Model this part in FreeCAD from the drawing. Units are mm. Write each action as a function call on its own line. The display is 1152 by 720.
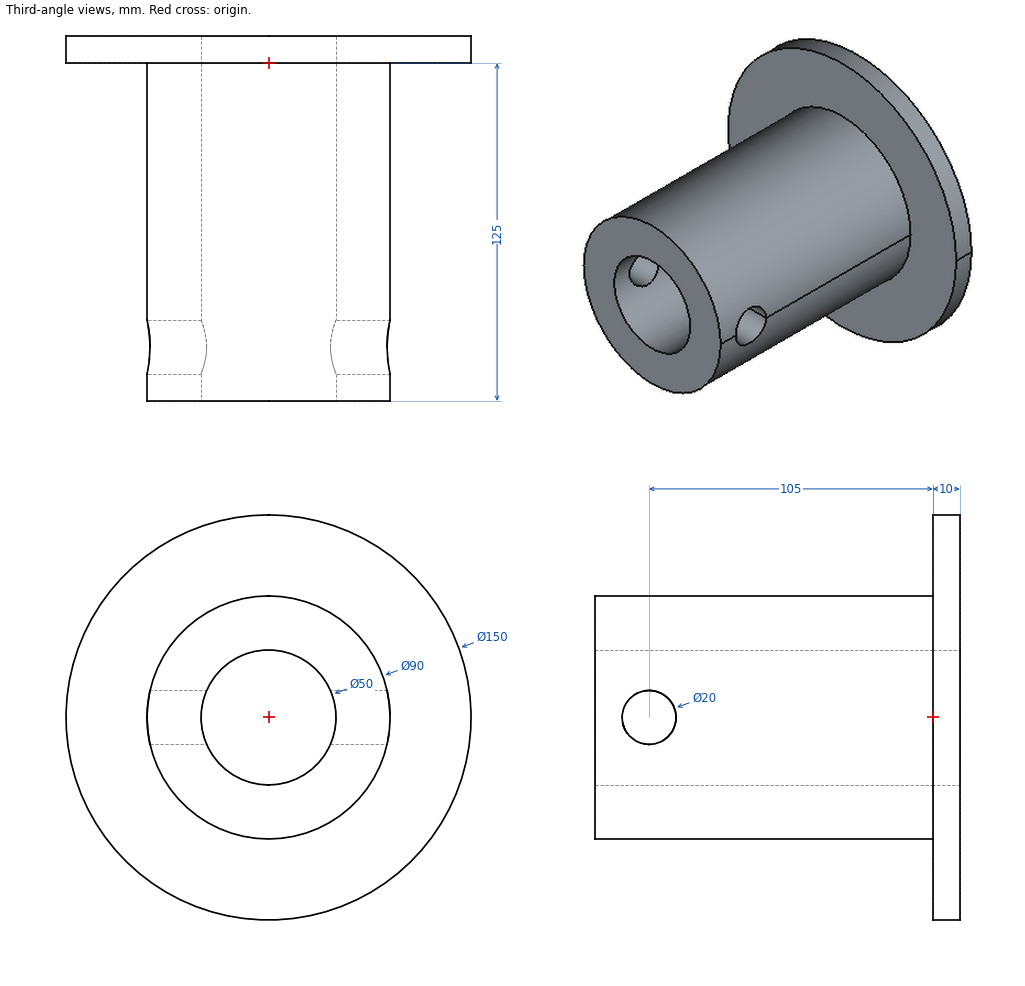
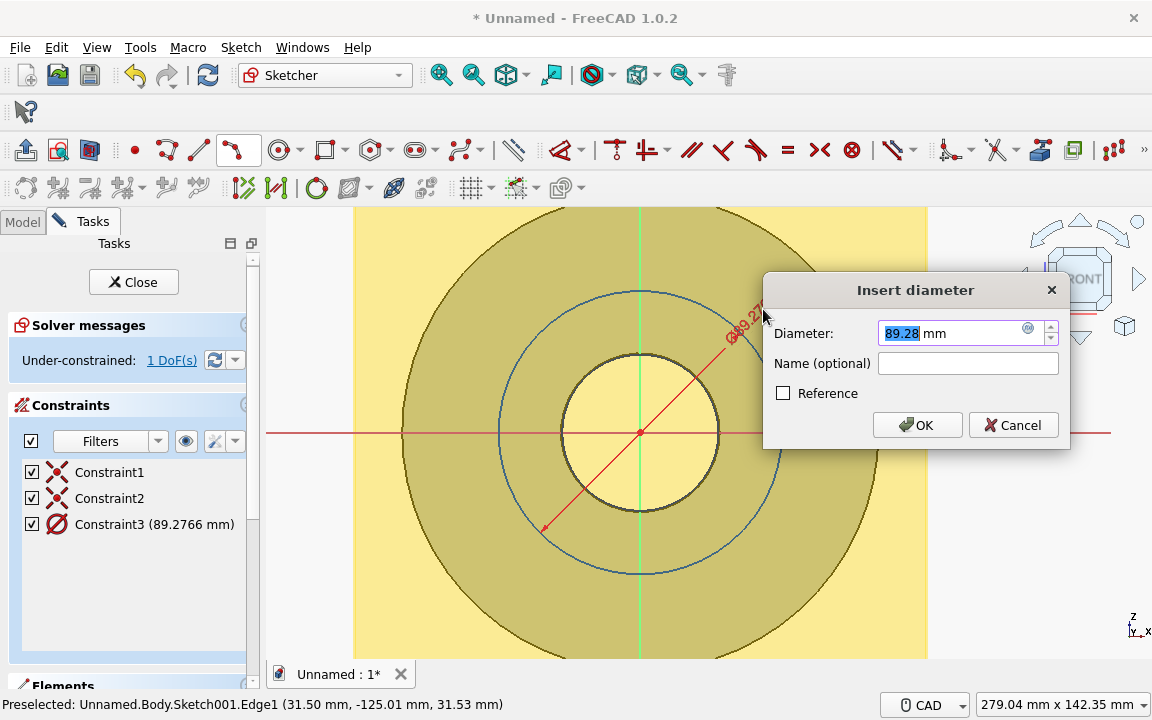
text(90)
key(Return)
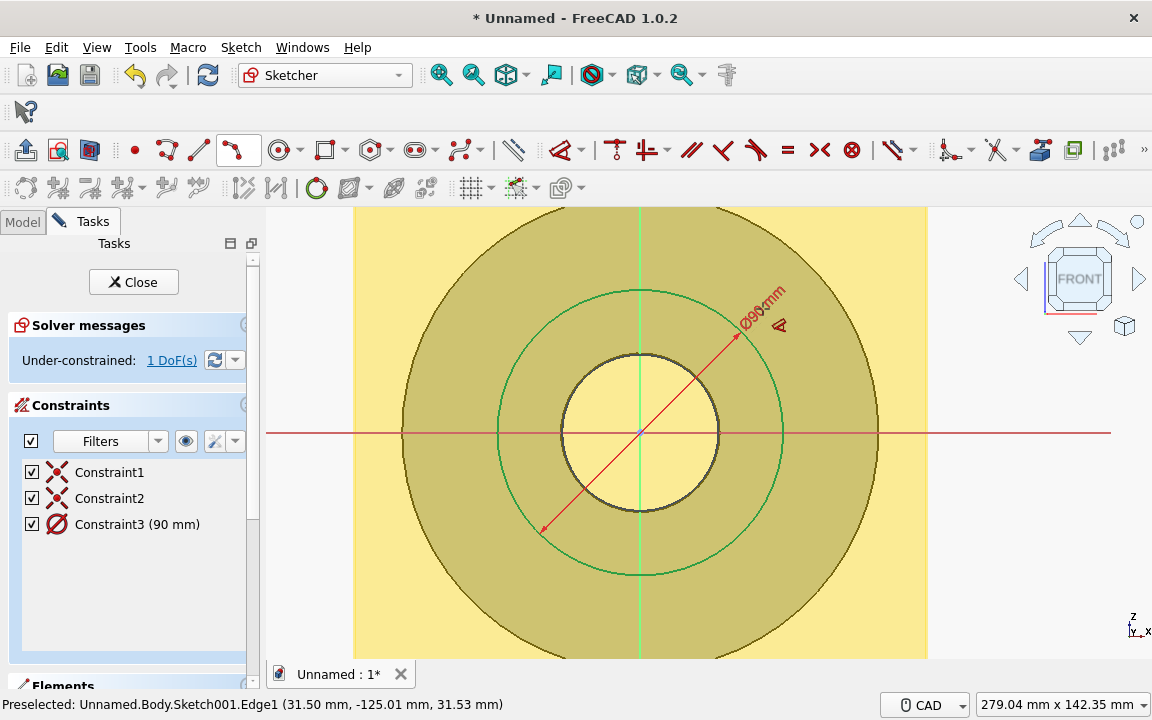
click(695, 377)
click(717, 354)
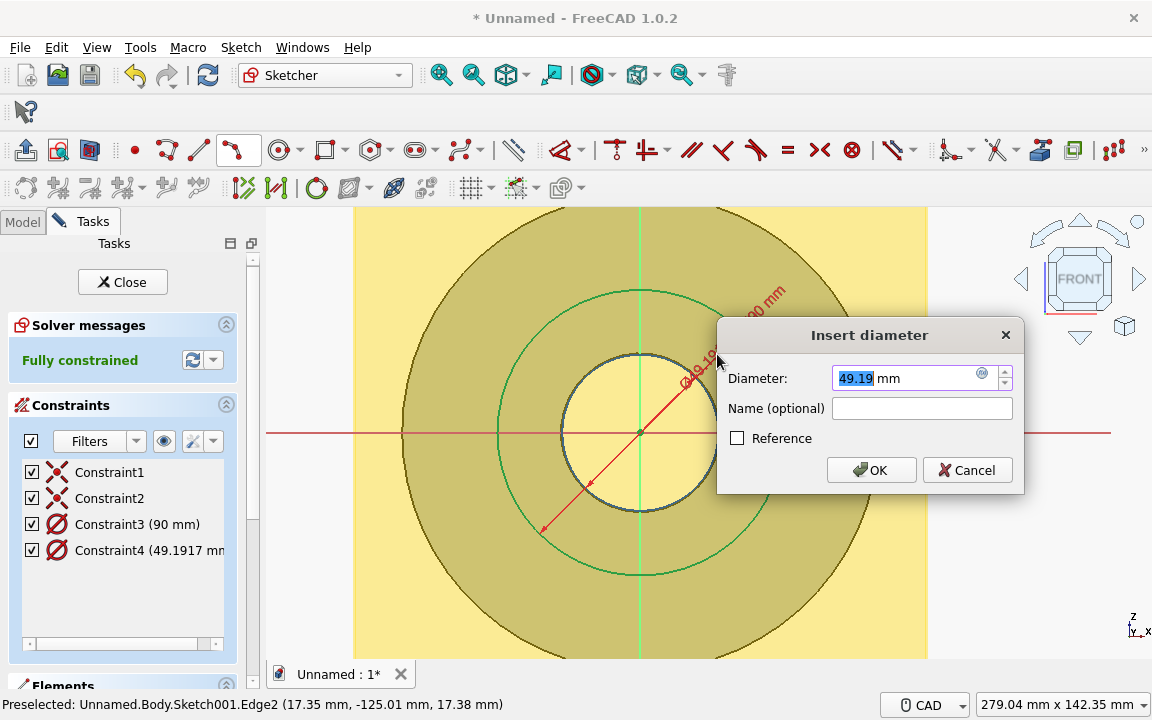
text(50)
key(Return)
key(Escape)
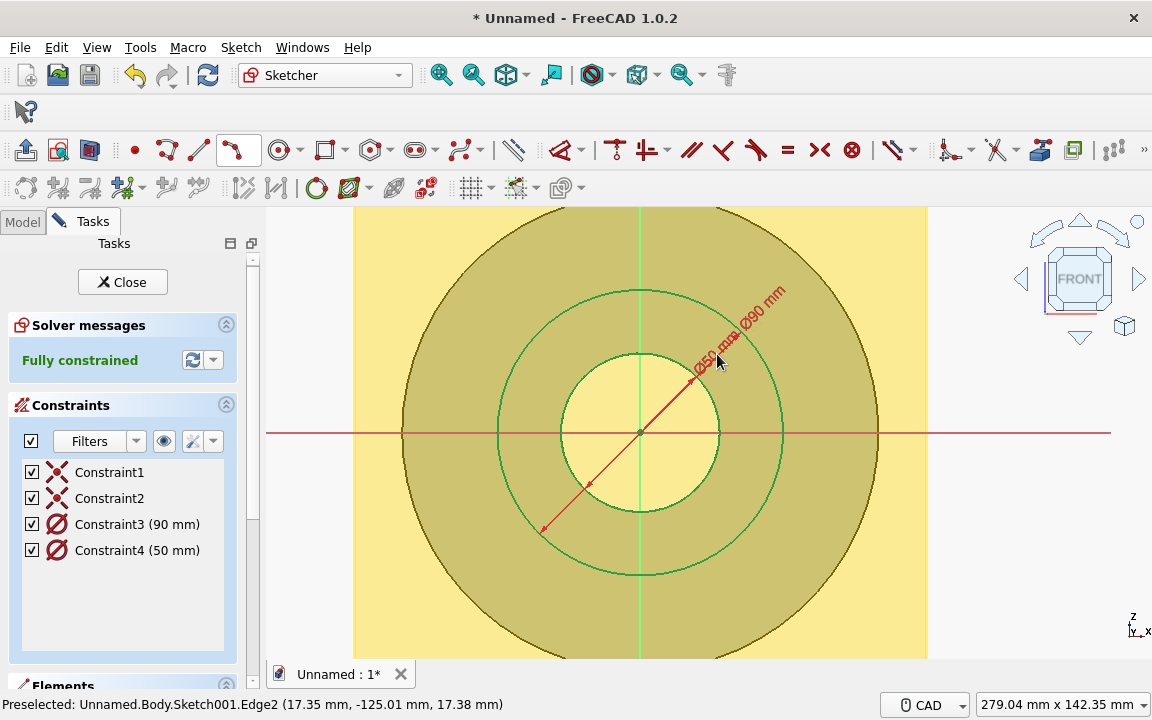
click(123, 282)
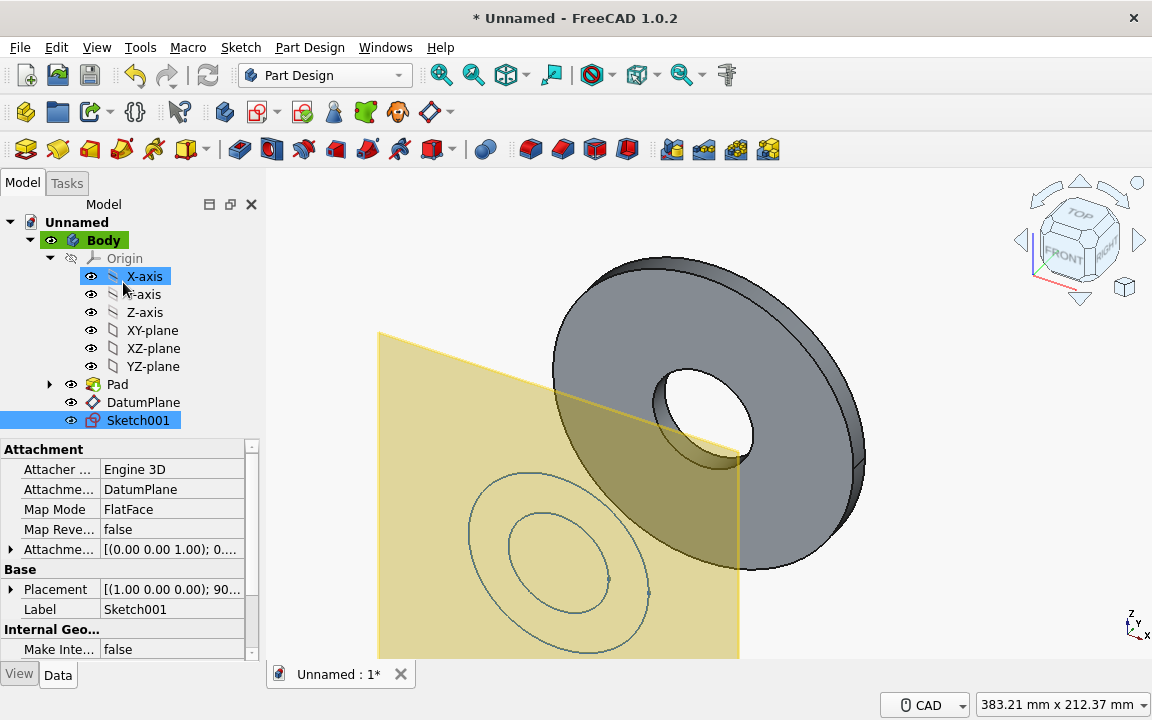
click(26, 150)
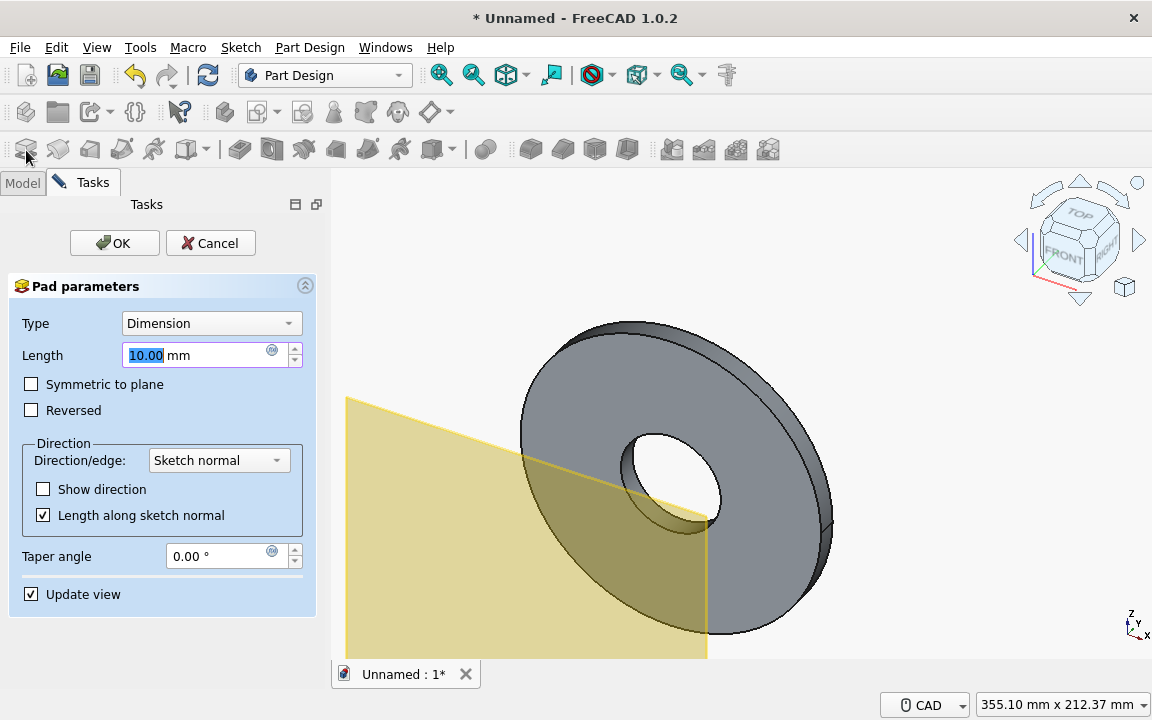
text(125)
key(Tab)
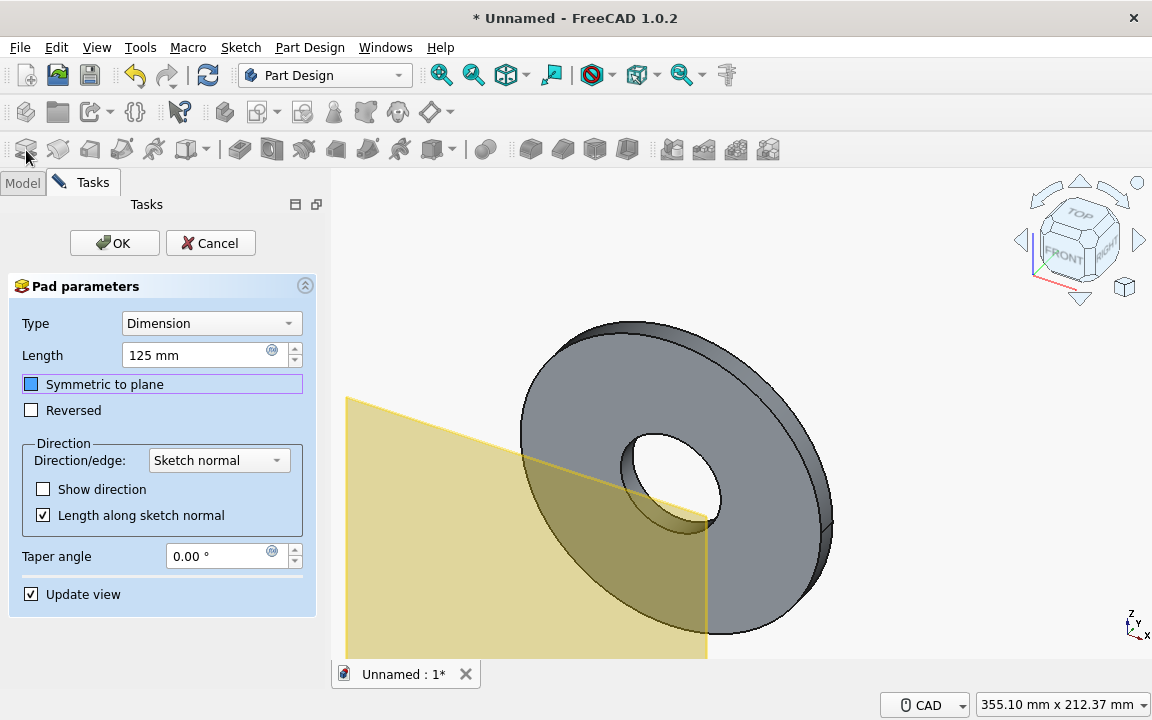
click(30, 410)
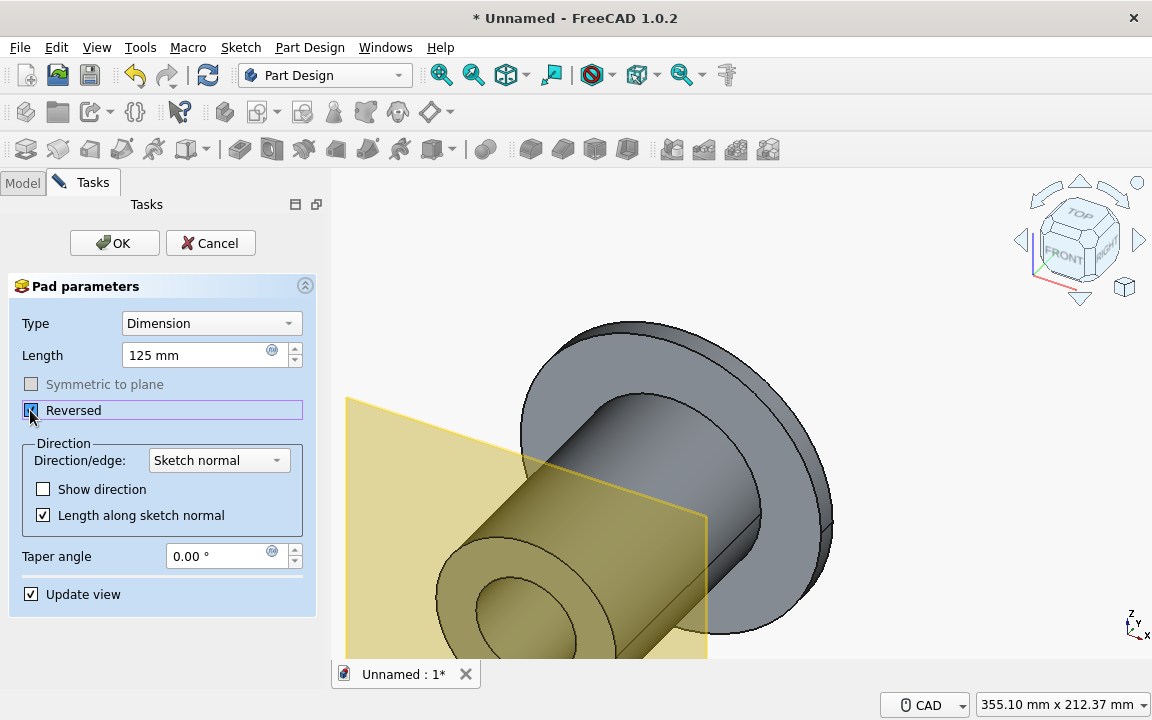
click(115, 243)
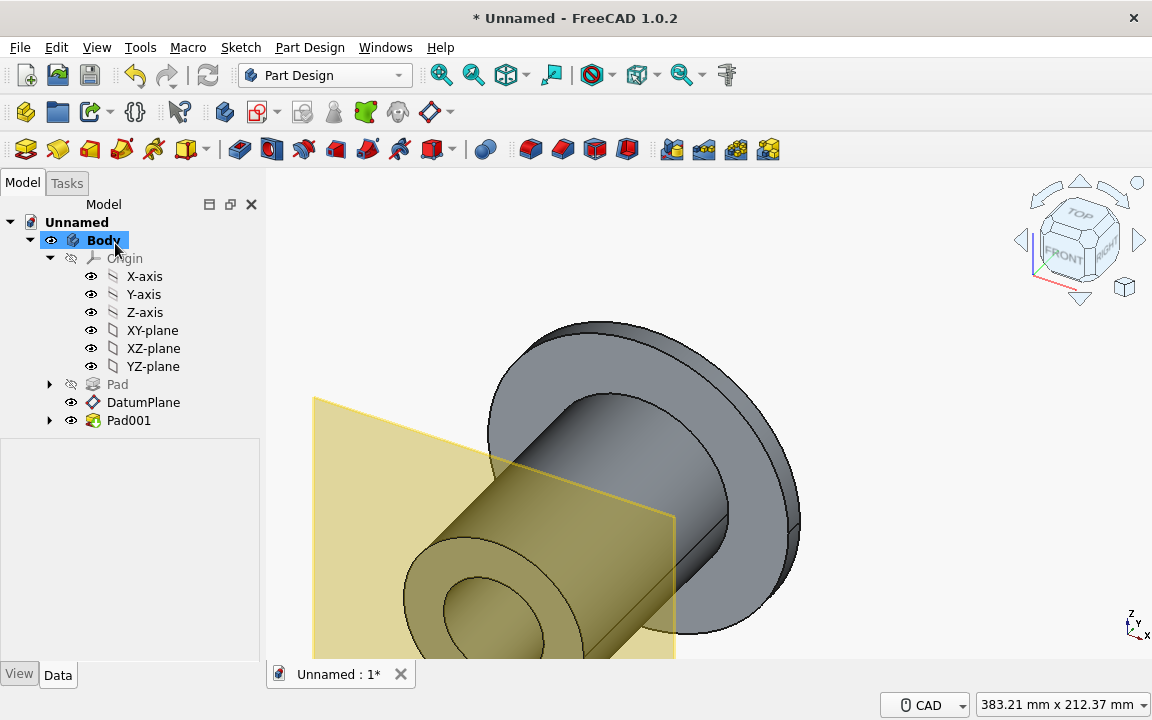
click(116, 402)
key(space)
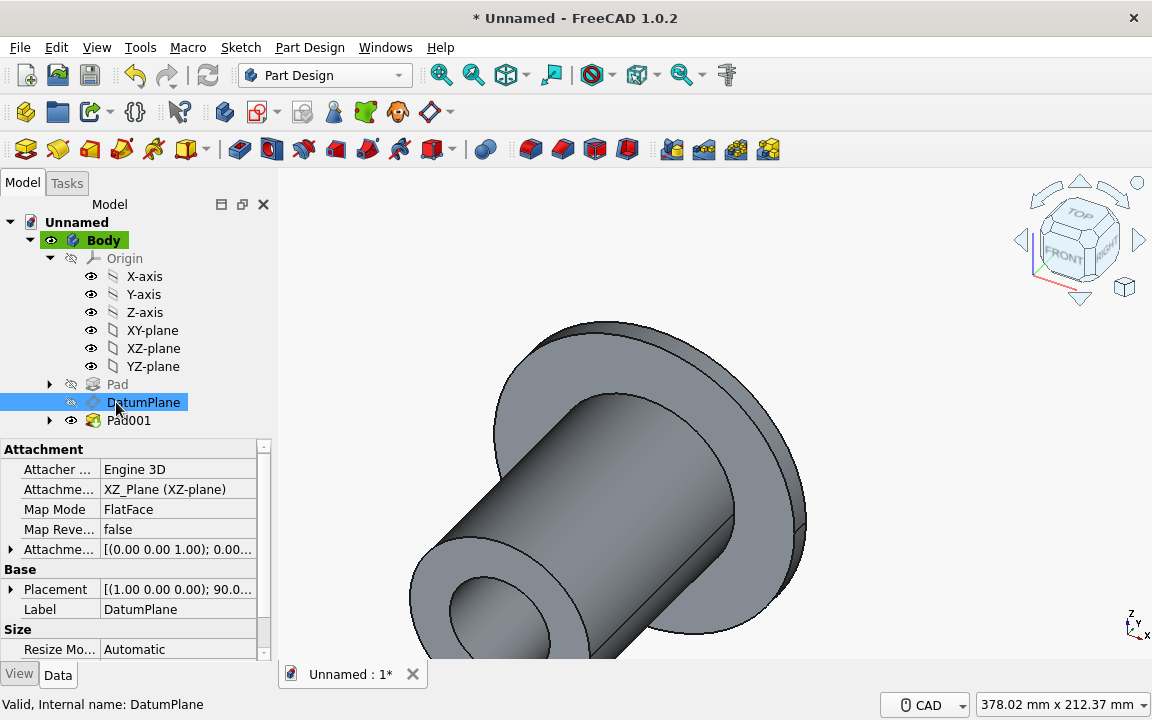
click(442, 76)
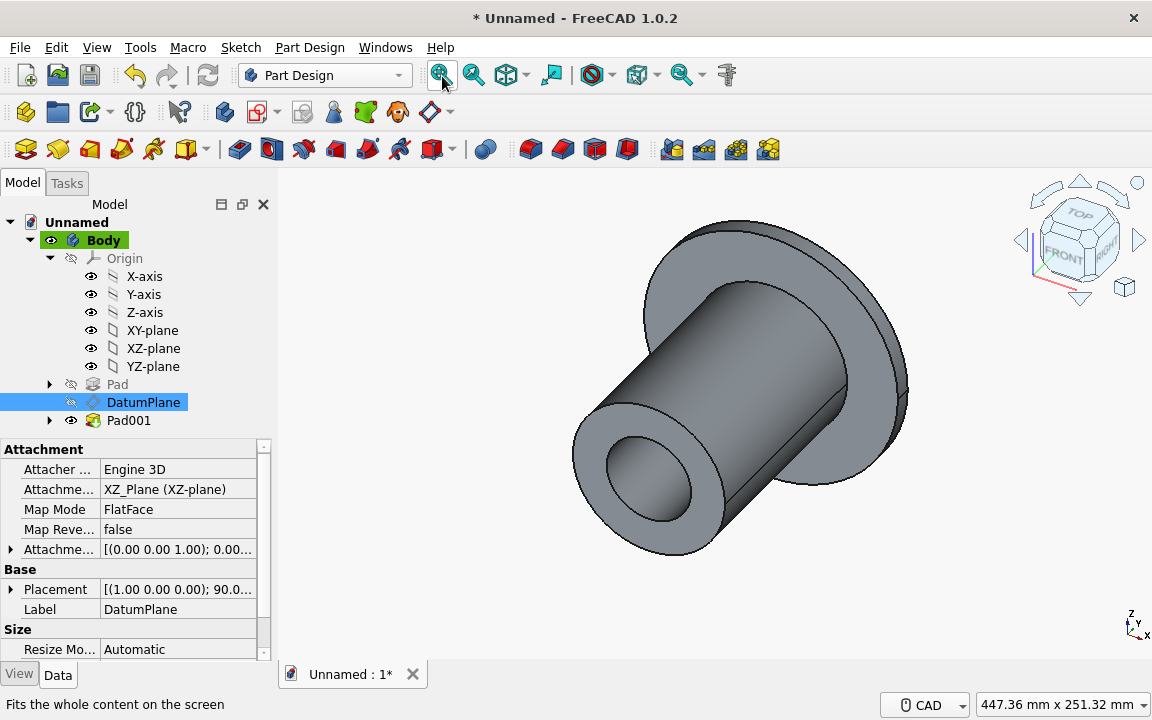
click(318, 619)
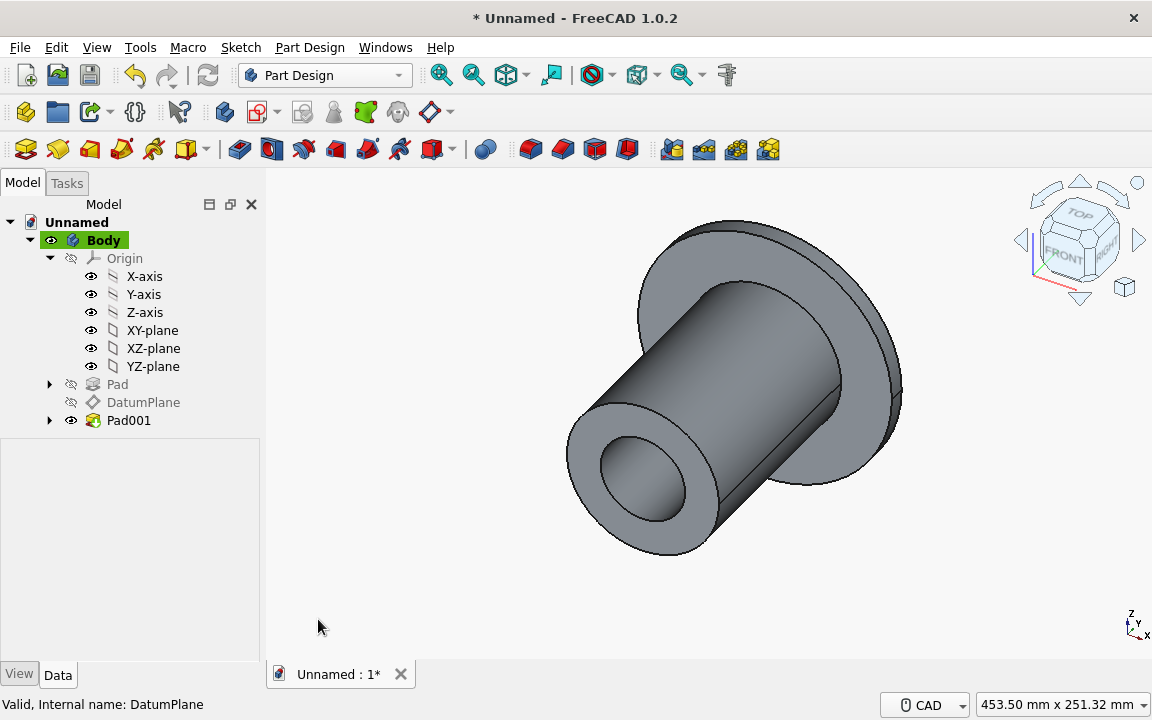
click(258, 112)